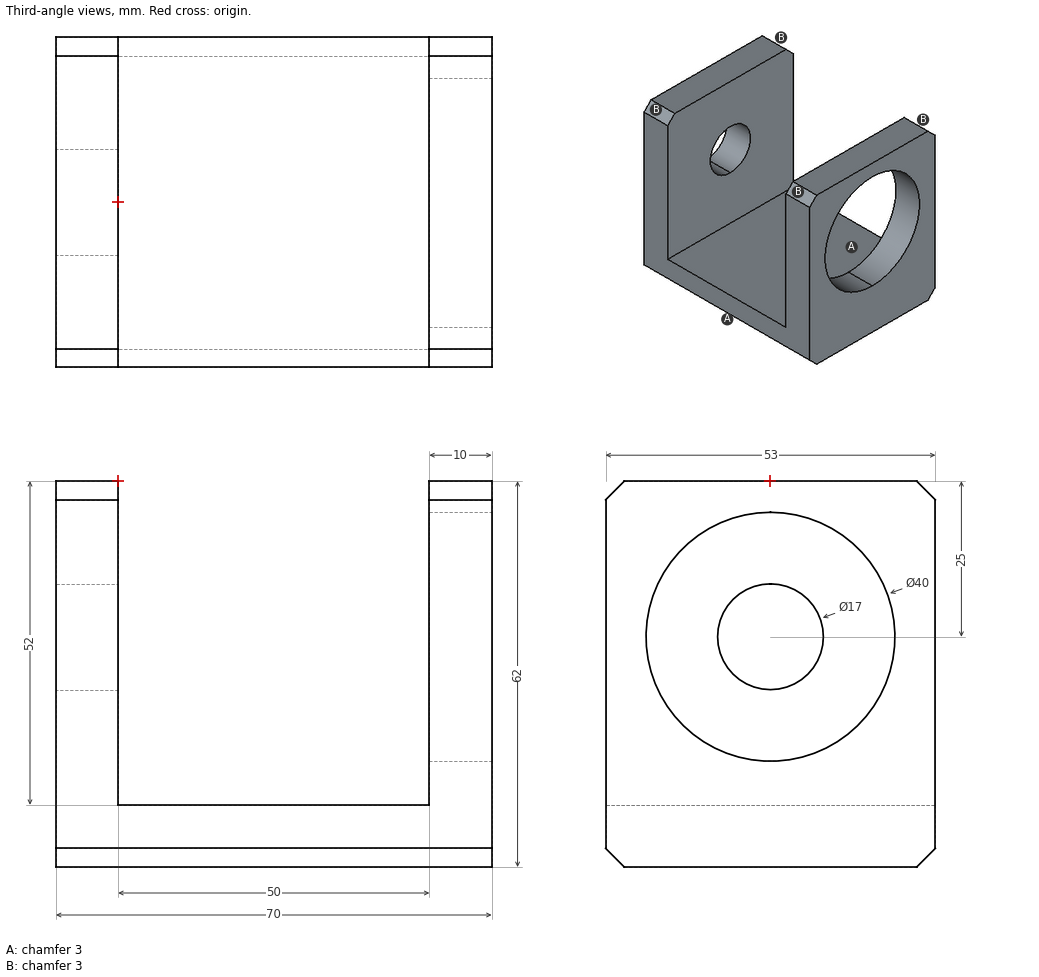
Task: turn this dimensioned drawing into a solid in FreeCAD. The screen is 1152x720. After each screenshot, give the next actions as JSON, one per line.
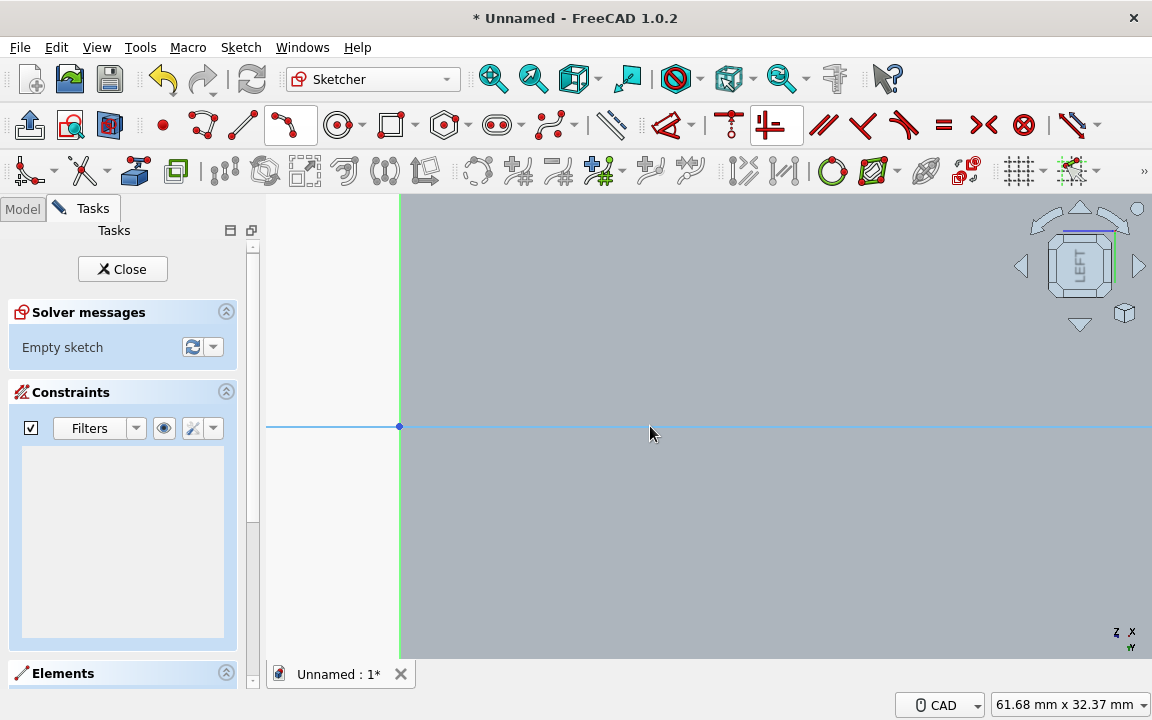
{"action": "left_click", "coordinate": [338, 126]}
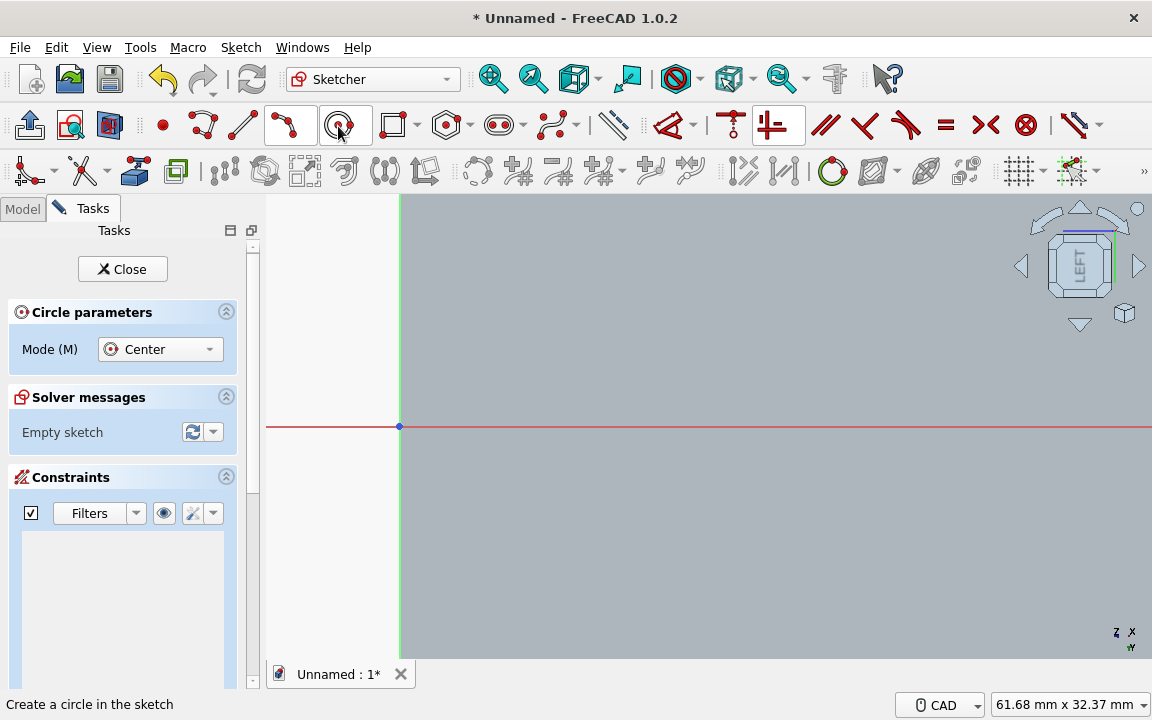
{"action": "left_click", "coordinate": [759, 426]}
{"action": "left_click", "coordinate": [845, 340]}
{"action": "key", "text": "Escape"}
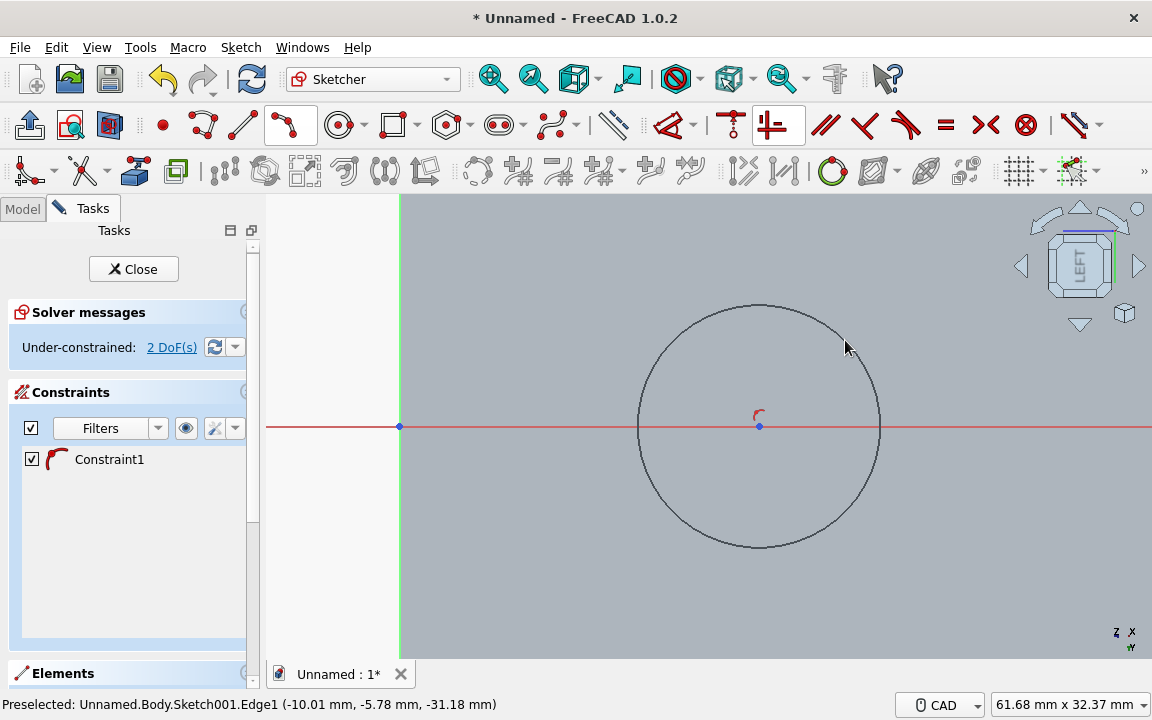
{"action": "key", "text": "d"}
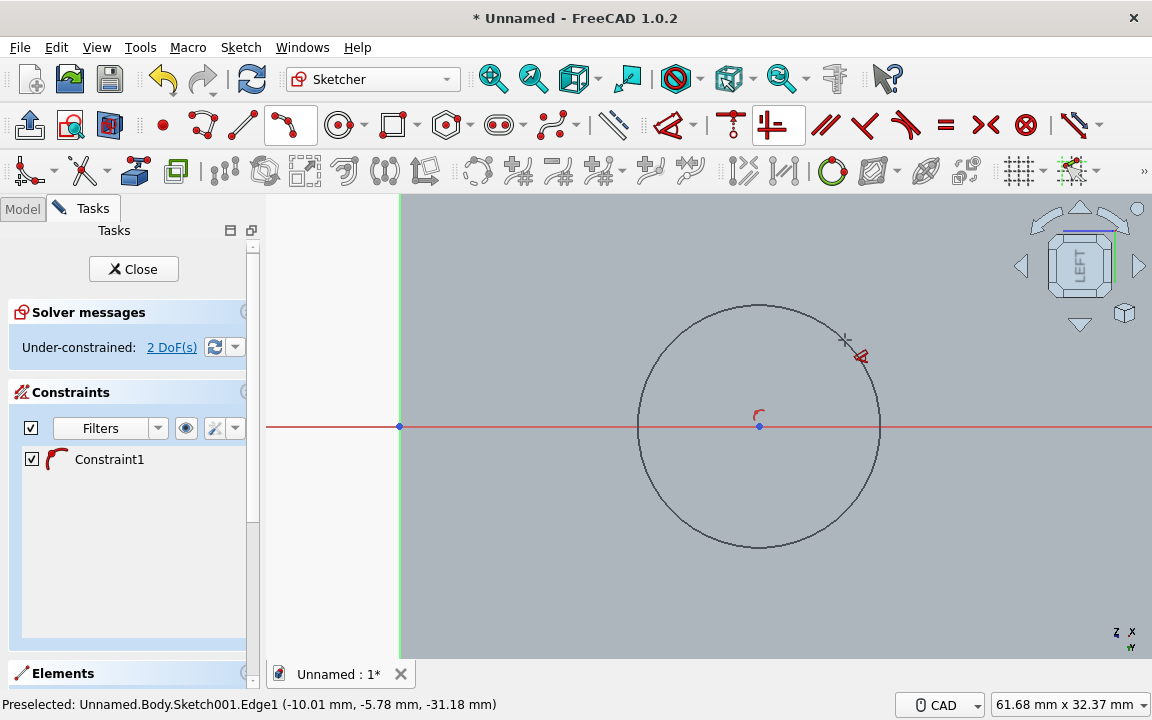
{"action": "left_click", "coordinate": [844, 340]}
{"action": "left_click", "coordinate": [866, 317]}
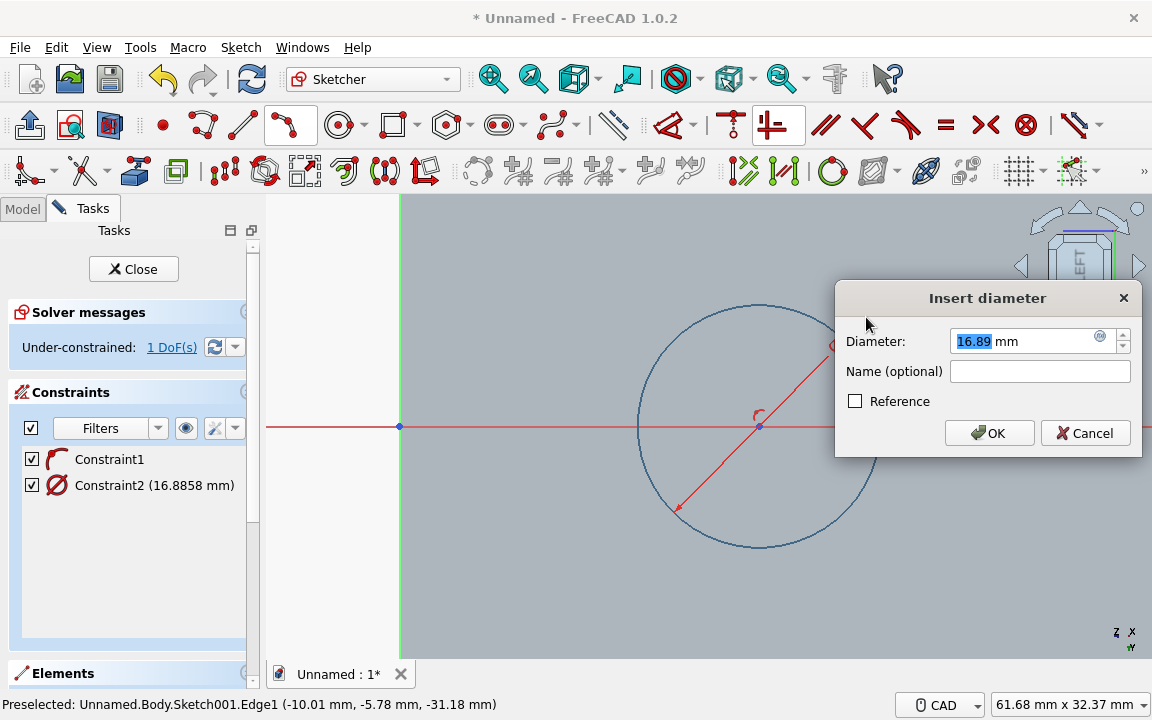
{"action": "type", "text": "17"}
{"action": "key", "text": "Return"}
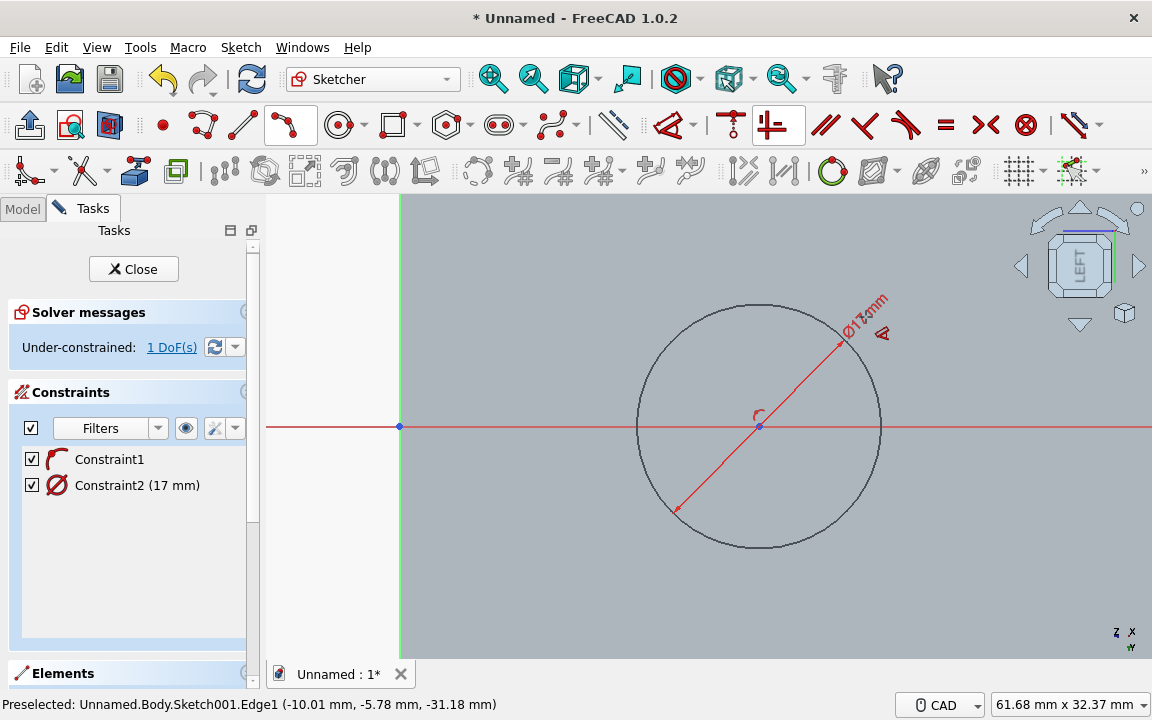
{"action": "left_click", "coordinate": [759, 426]}
{"action": "left_click", "coordinate": [579, 460]}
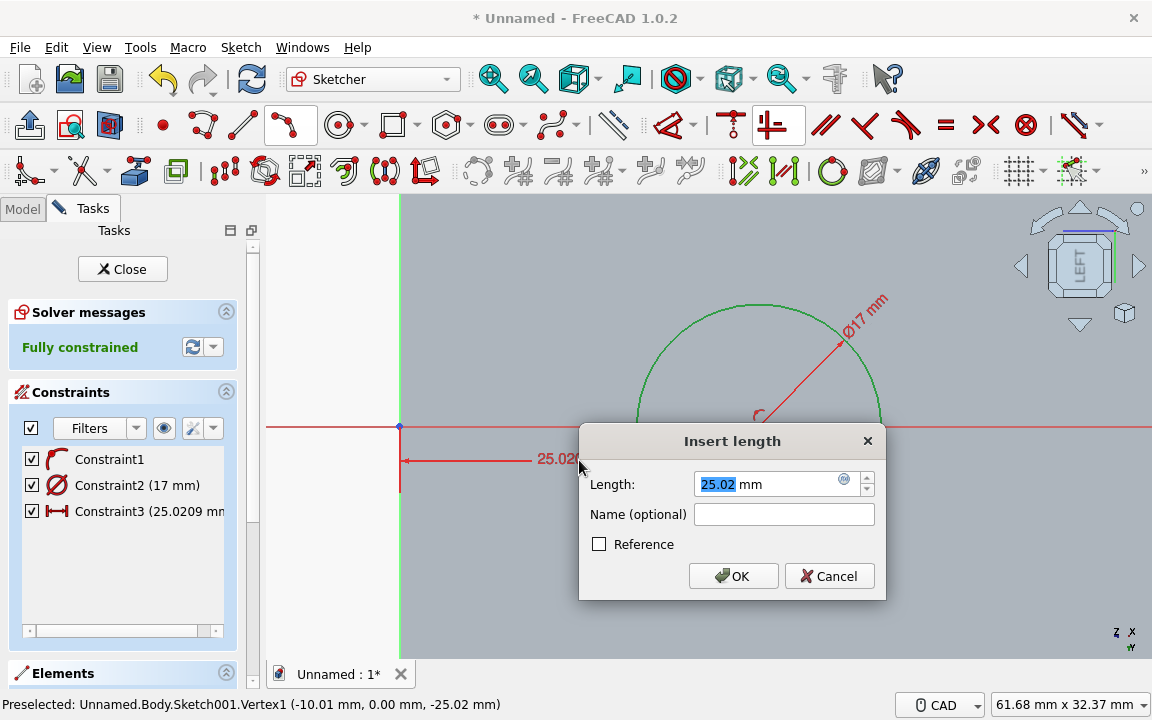
{"action": "type", "text": "25"}
{"action": "key", "text": "Return"}
{"action": "key", "text": "Escape"}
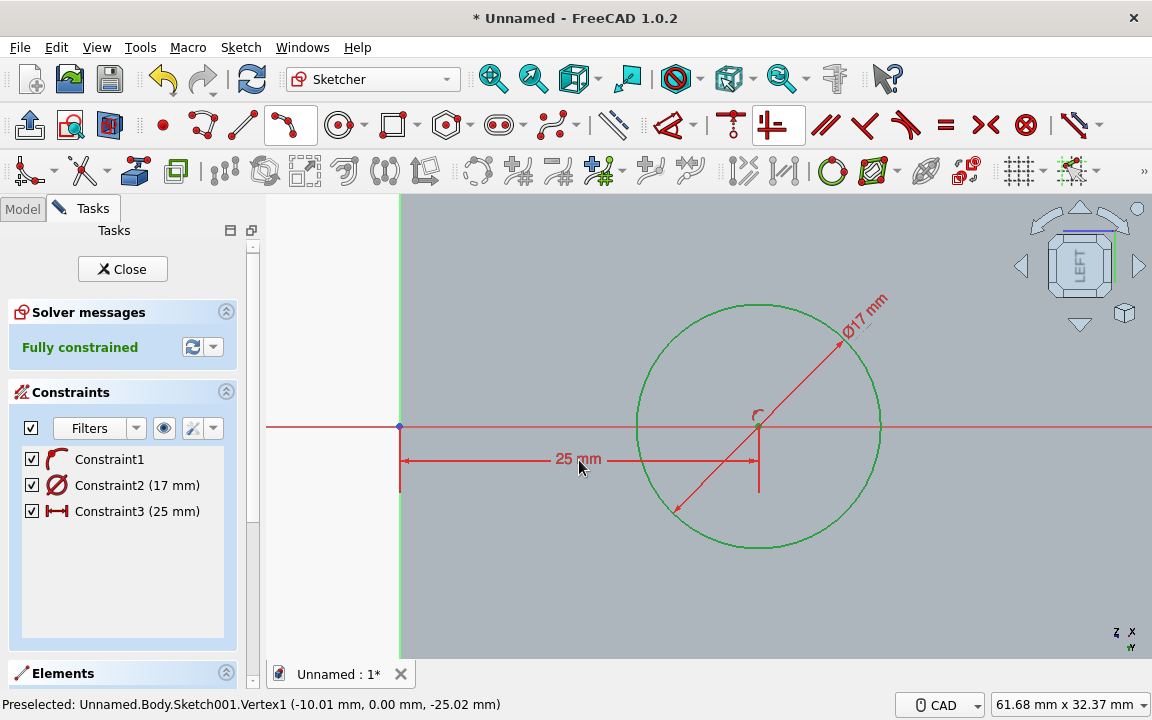
{"action": "left_click", "coordinate": [123, 269]}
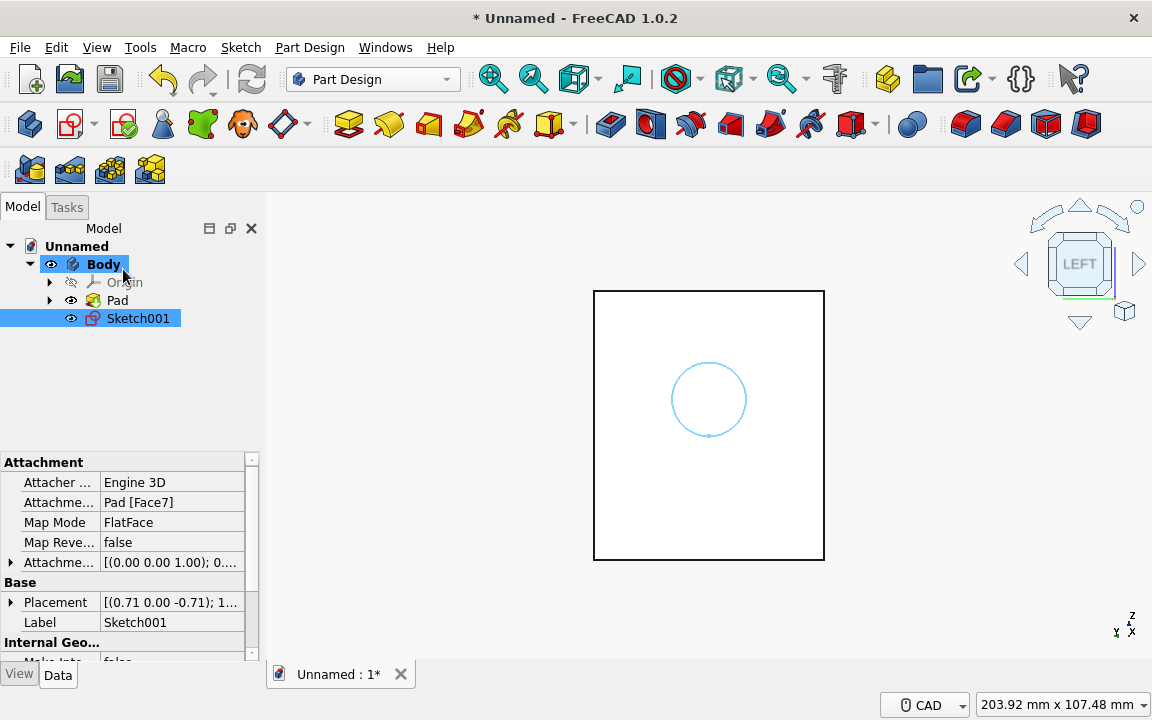
{"action": "left_click", "coordinate": [612, 124]}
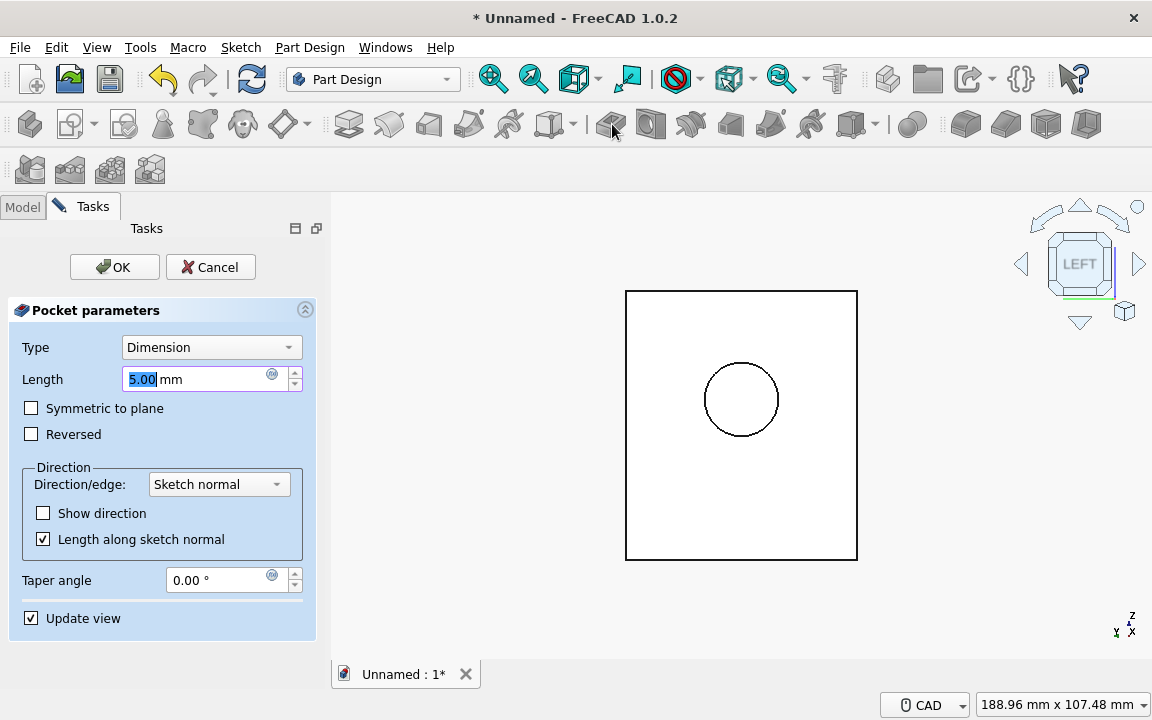
{"action": "left_click", "coordinate": [212, 348]}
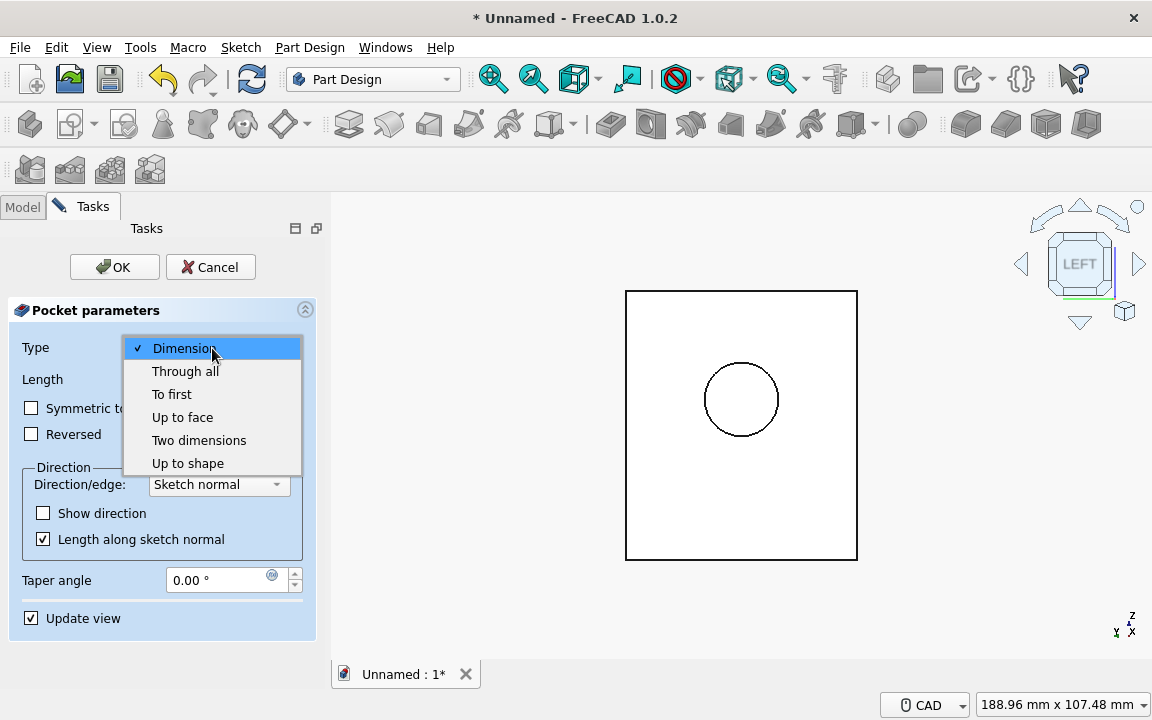
{"action": "left_click", "coordinate": [212, 394]}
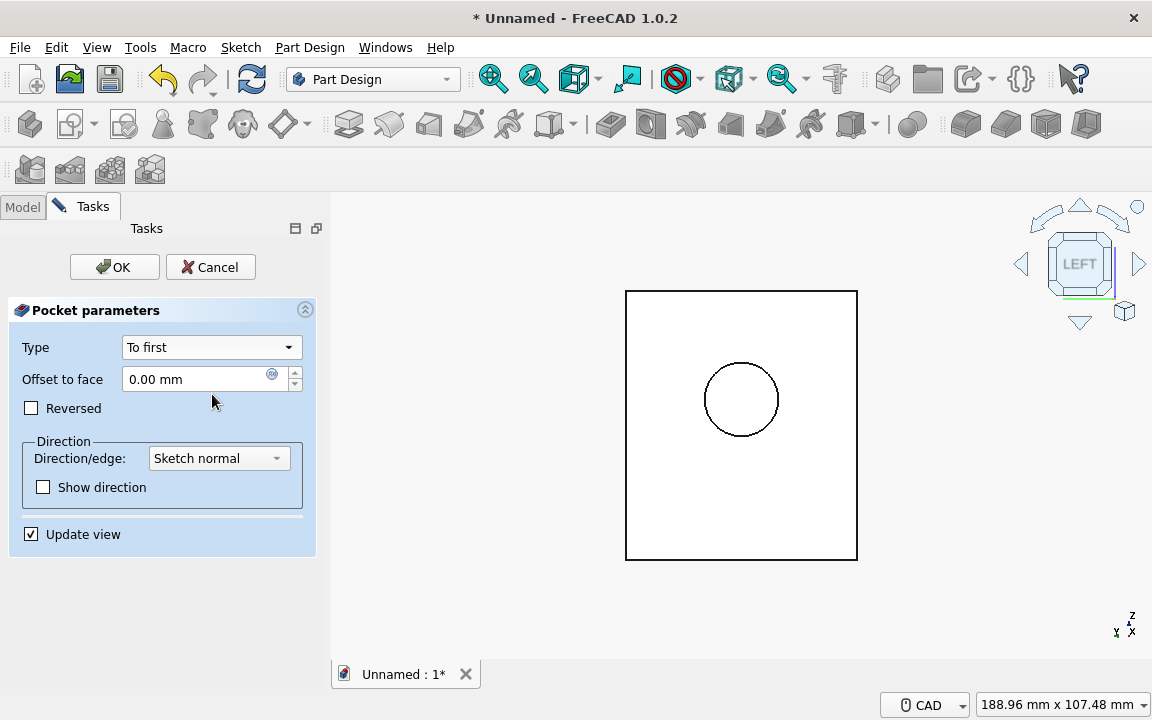
{"action": "left_click", "coordinate": [115, 267]}